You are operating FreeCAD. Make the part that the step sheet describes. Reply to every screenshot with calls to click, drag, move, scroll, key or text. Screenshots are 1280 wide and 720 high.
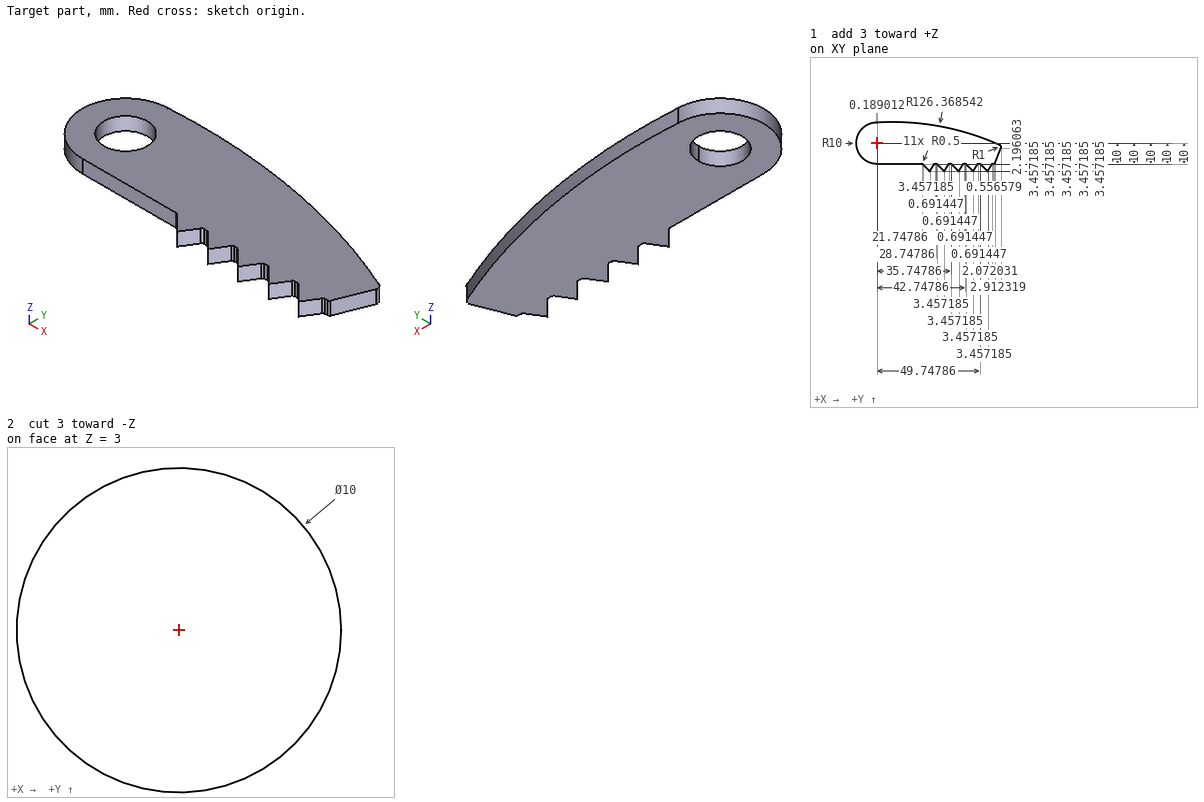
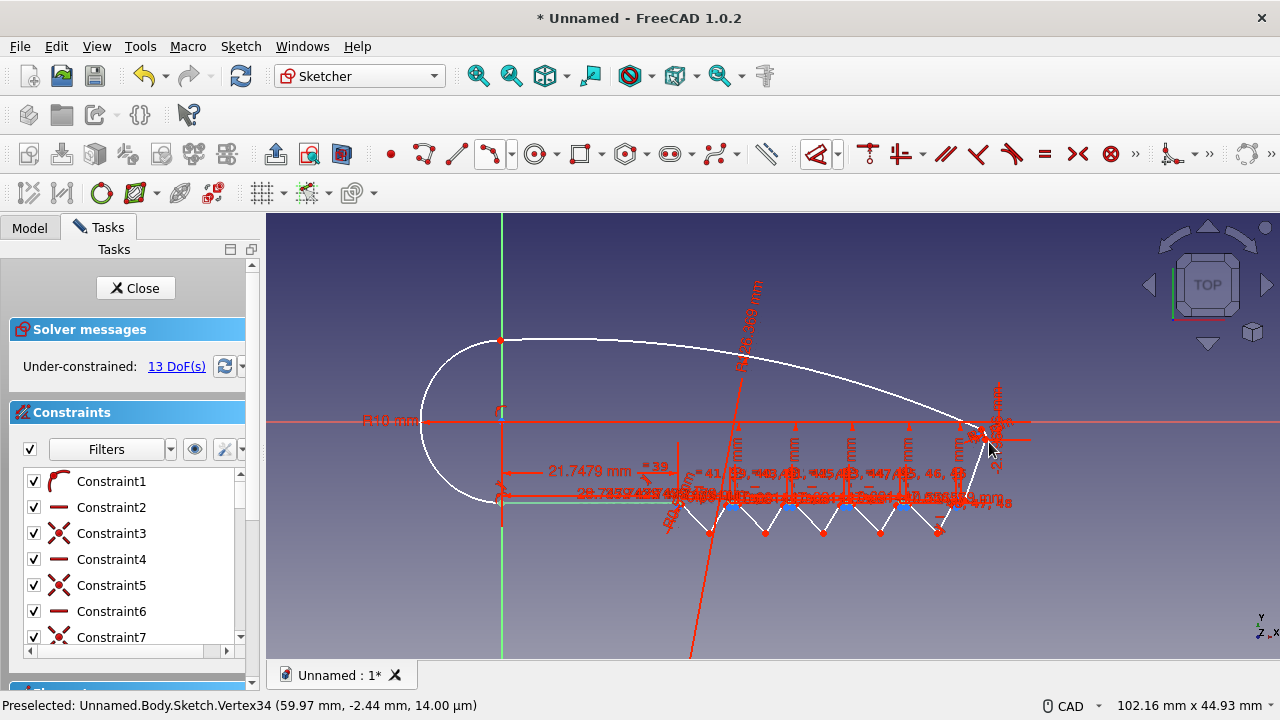
scroll(500, 341, up, 17)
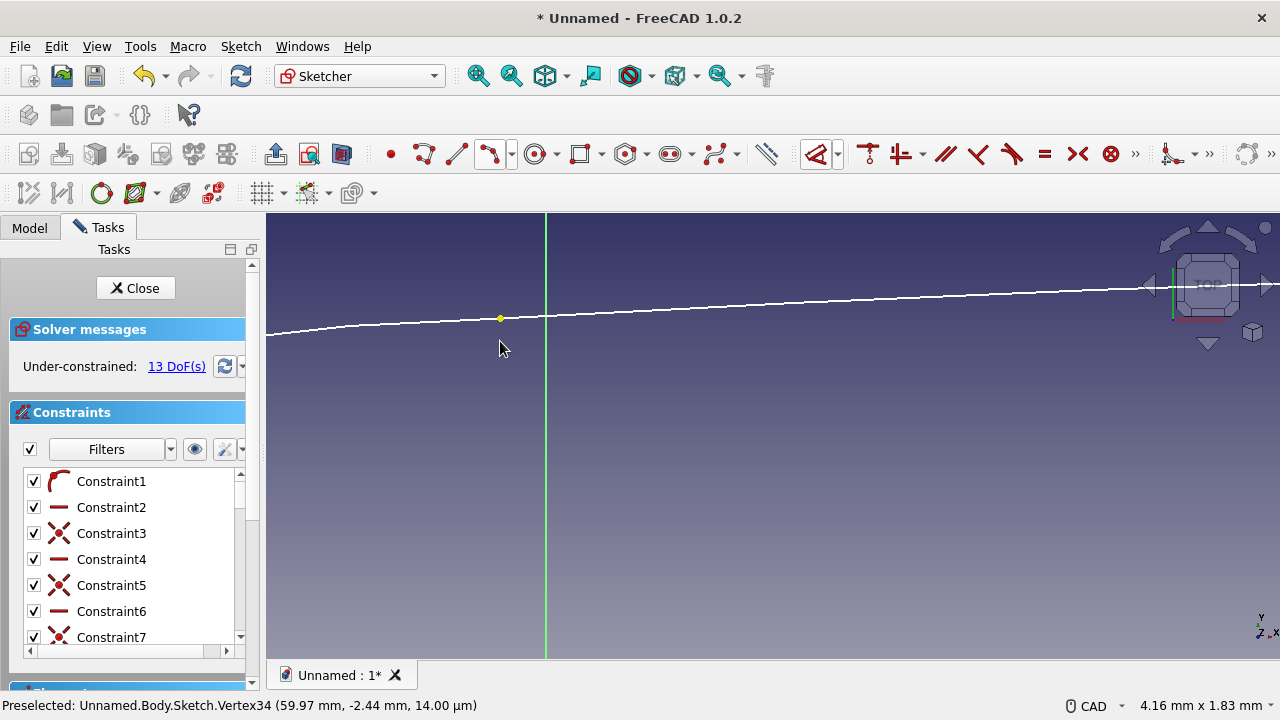
click(501, 318)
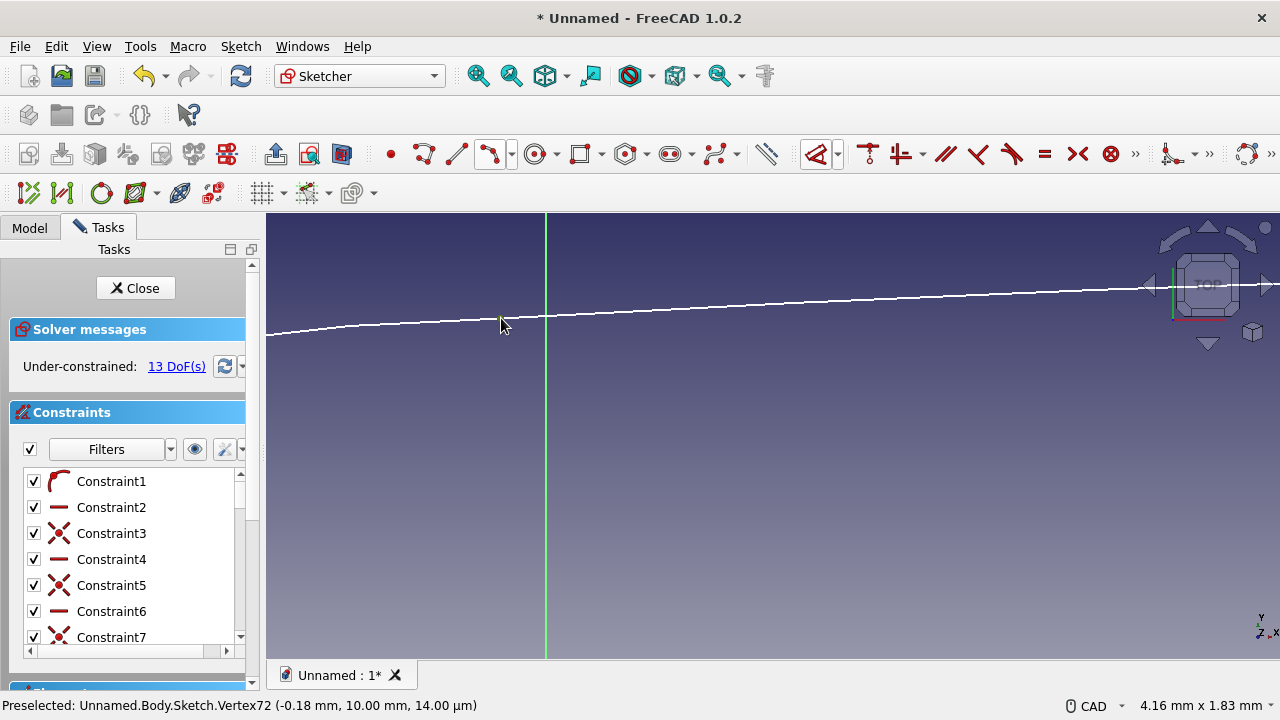
key(l)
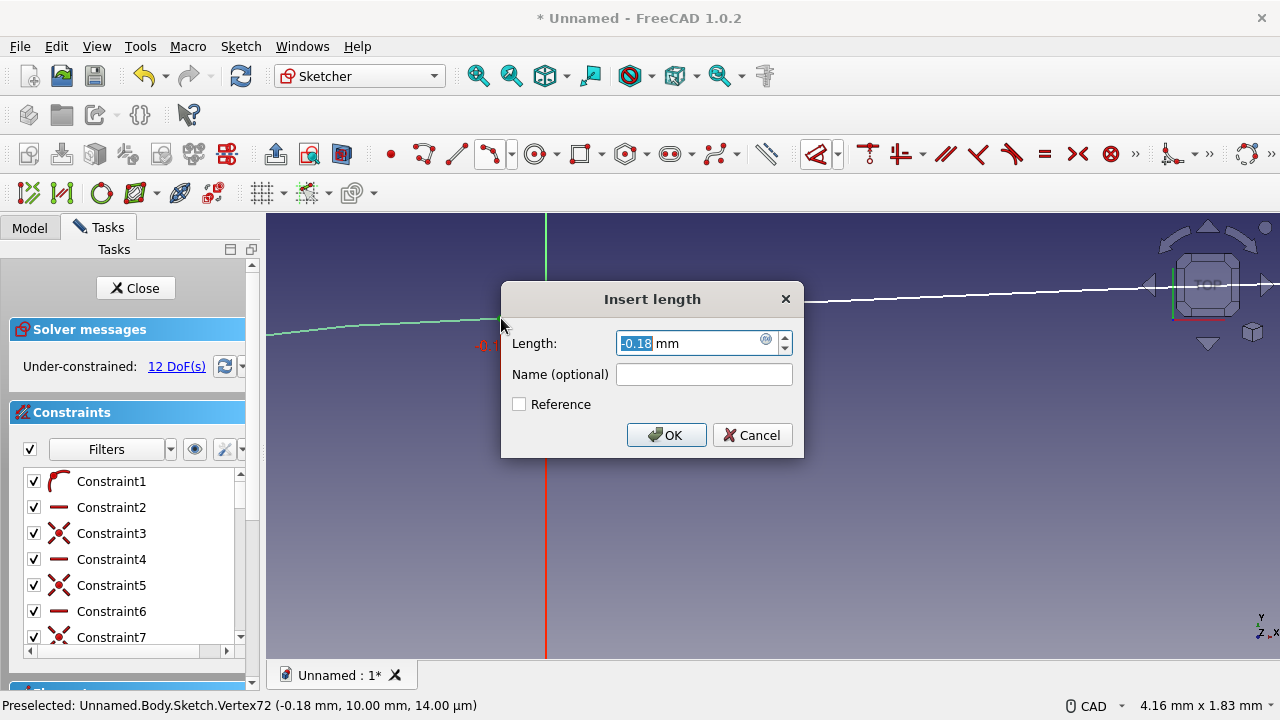
text(-0.189012)
key(Return)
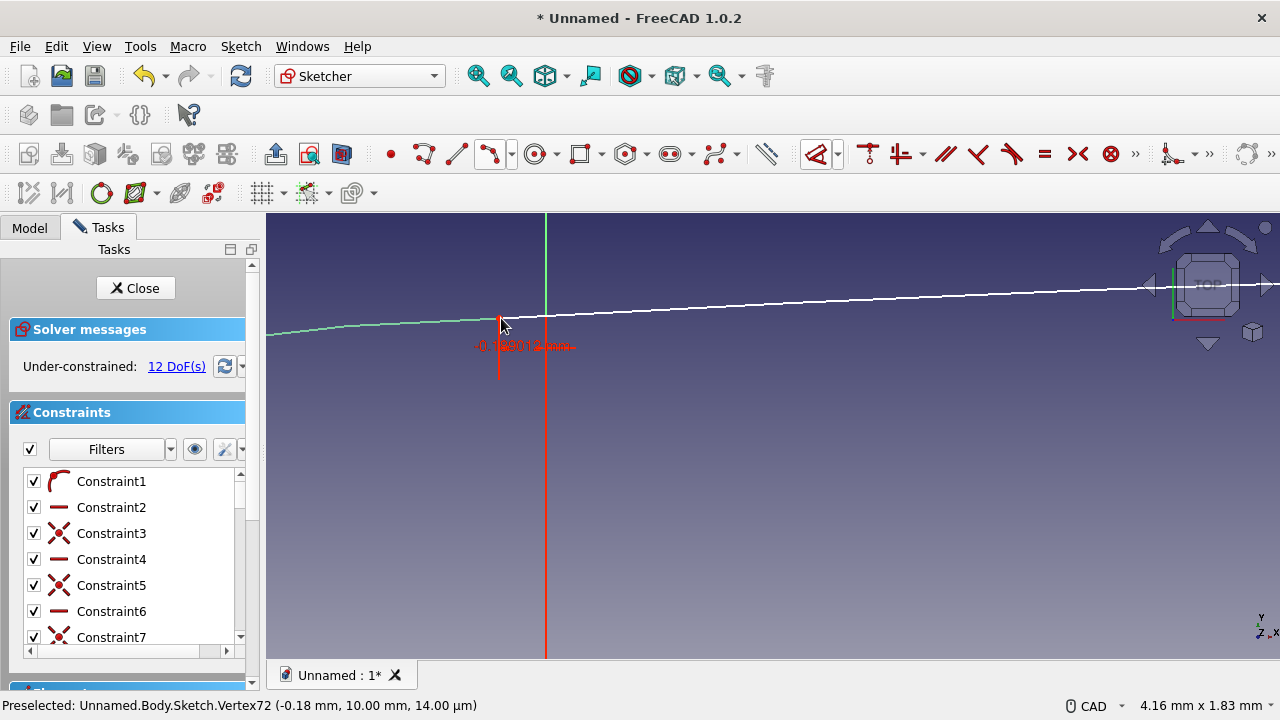
scroll(453, 319, down, 16)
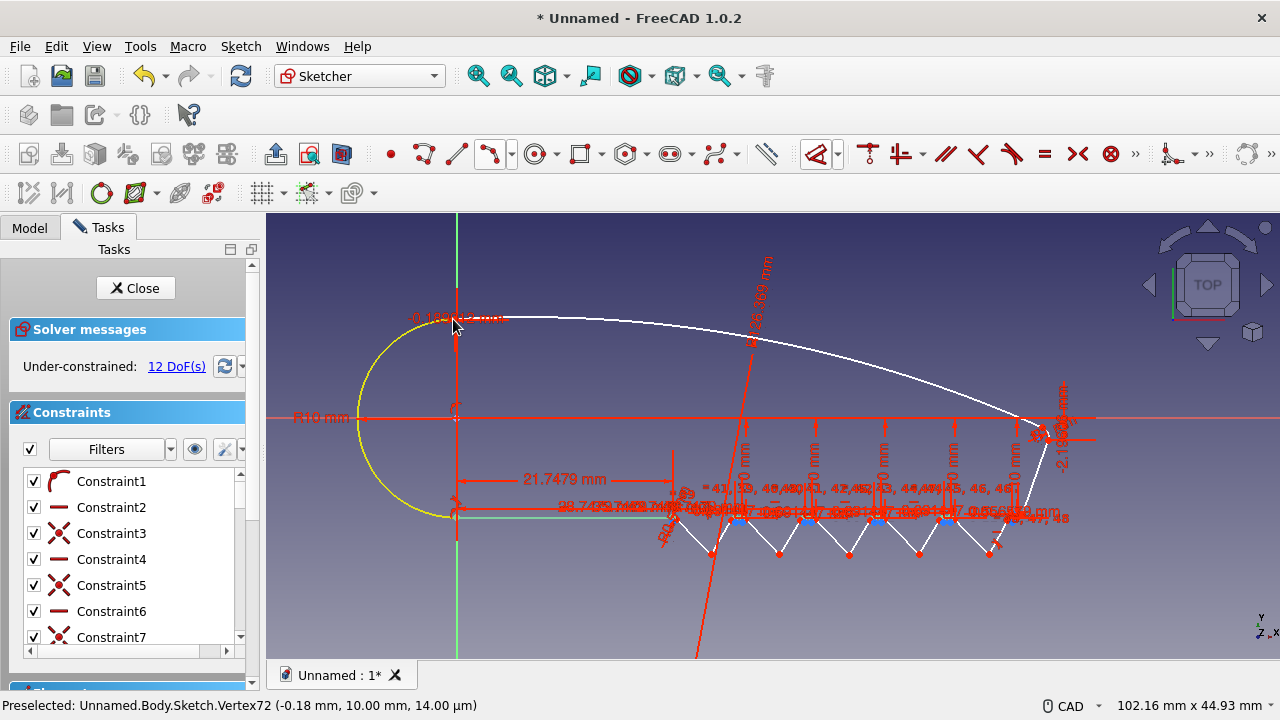
click(687, 530)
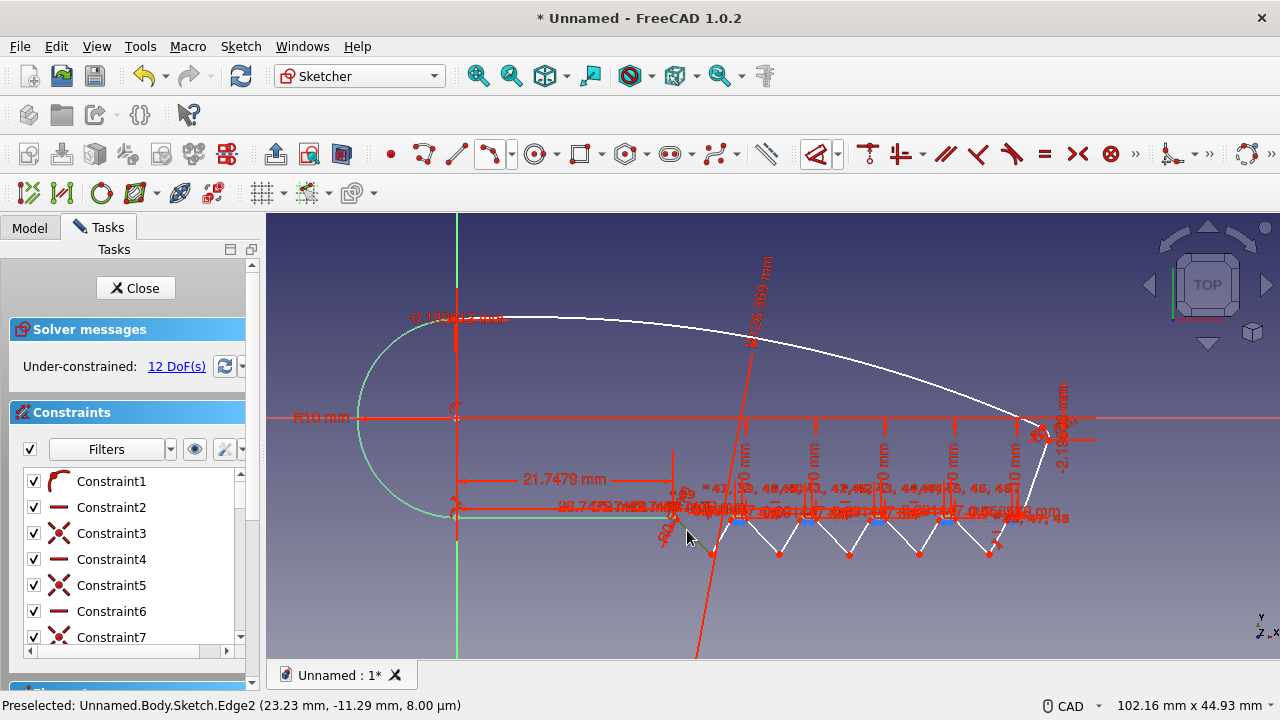
click(838, 154)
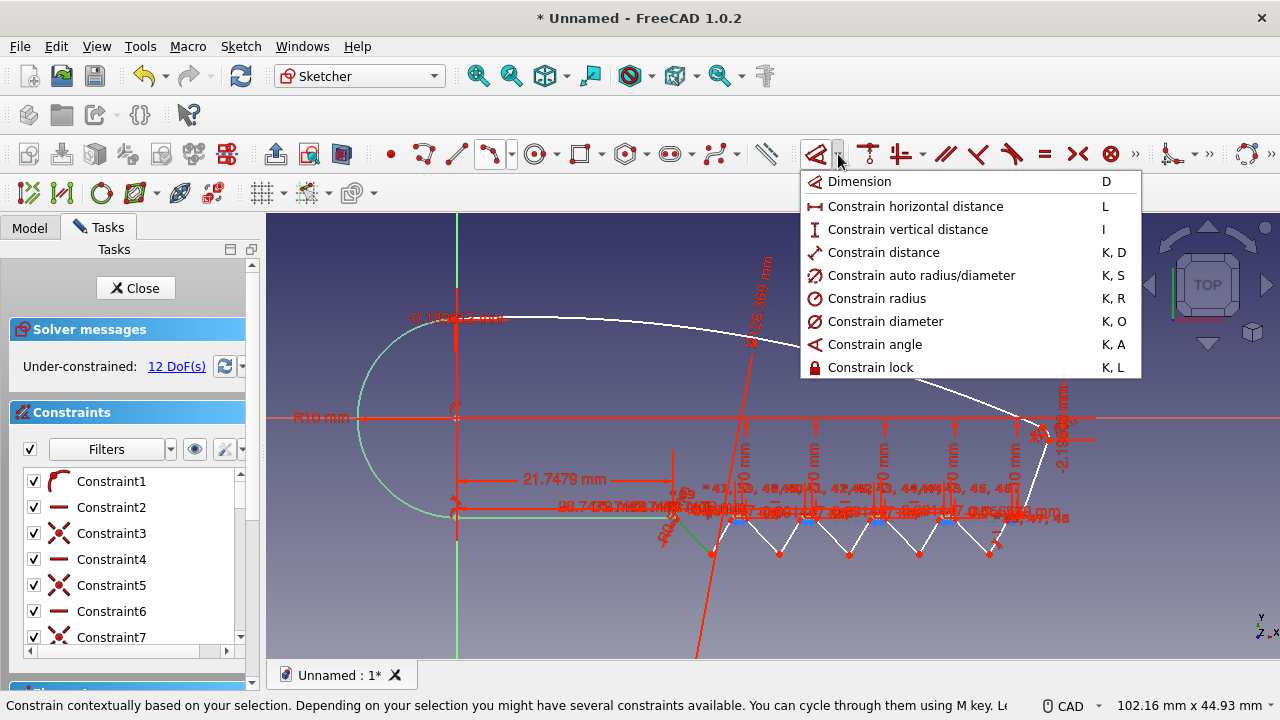
click(971, 206)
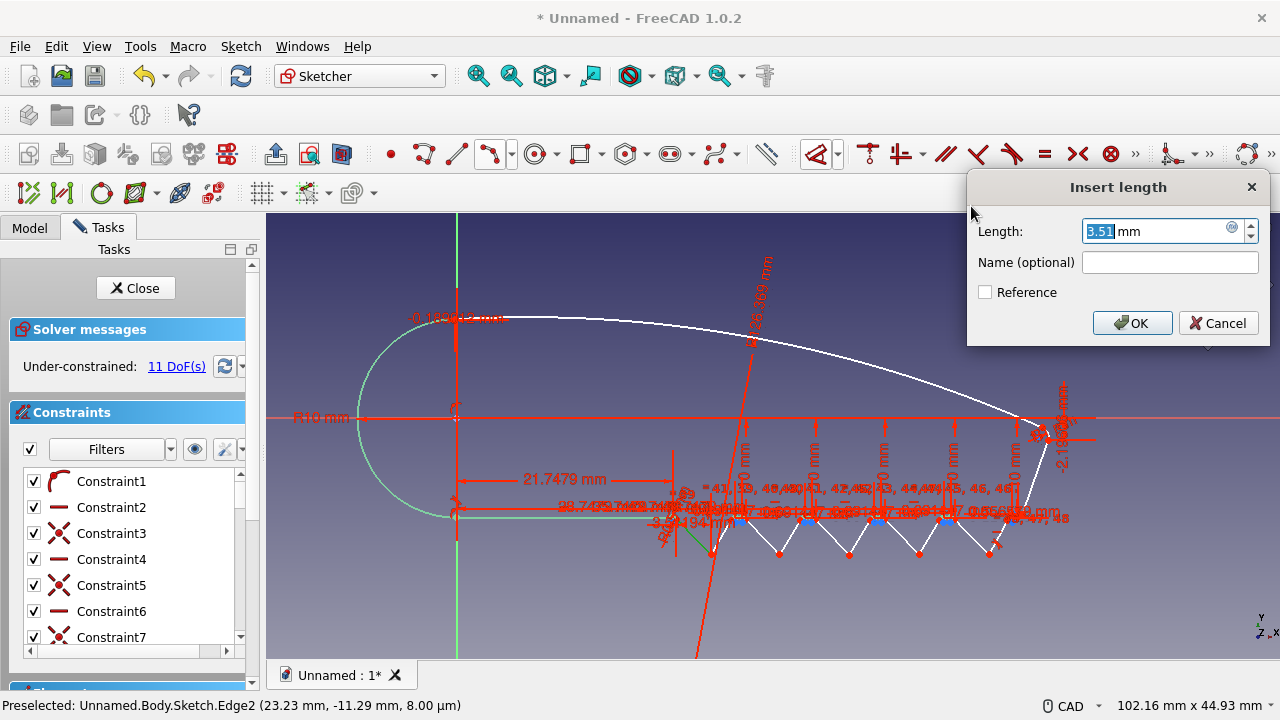
text(3.457185)
key(Return)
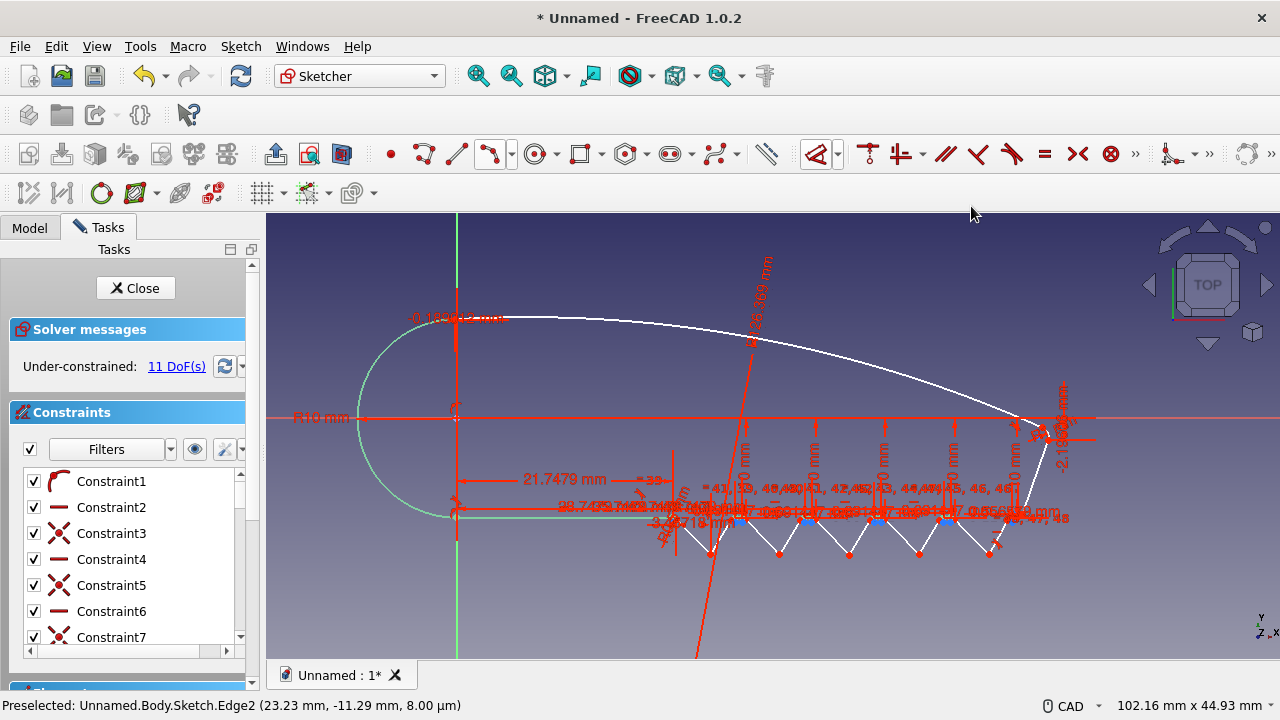
click(700, 544)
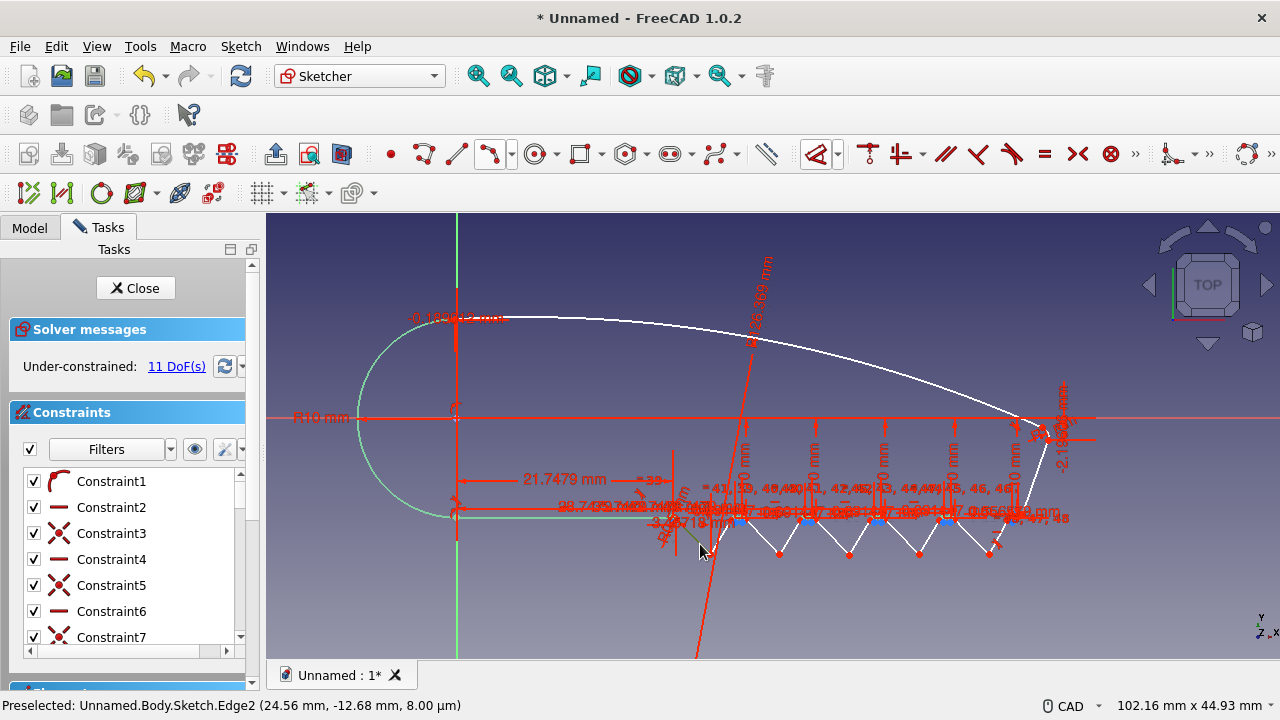
key(i)